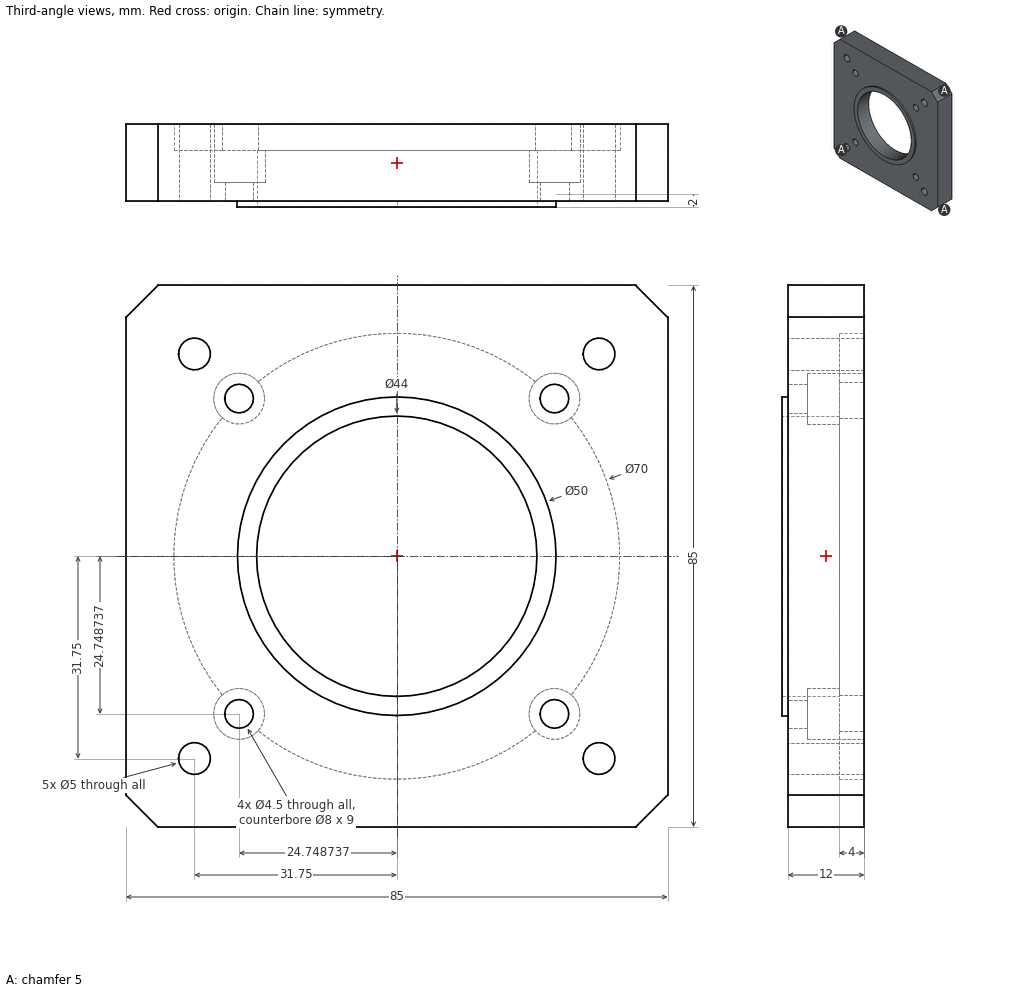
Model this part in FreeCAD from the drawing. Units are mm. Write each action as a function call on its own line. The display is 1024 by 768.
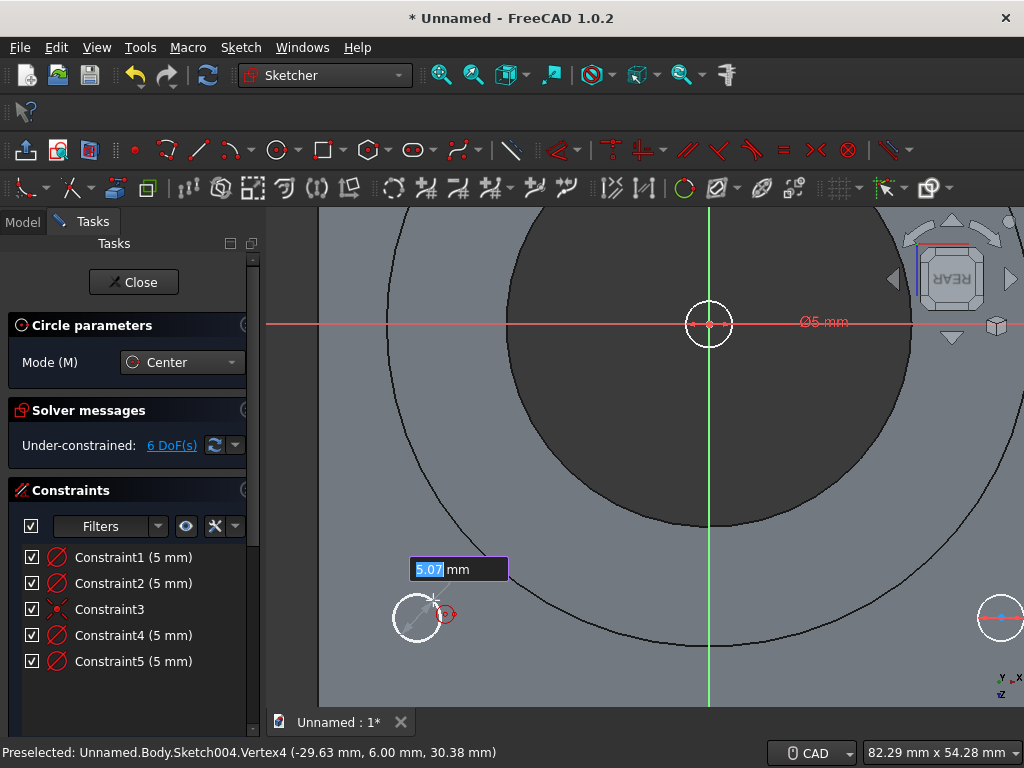
text(5)
key(Return)
key(Escape)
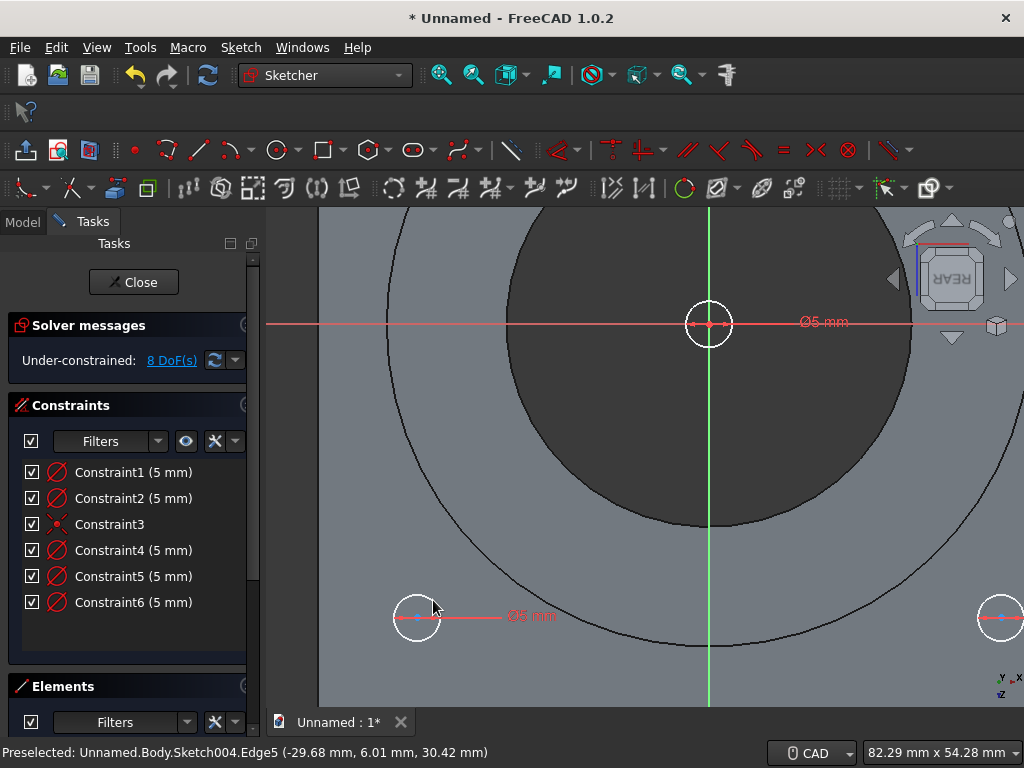
scroll(415, 618, down, 3)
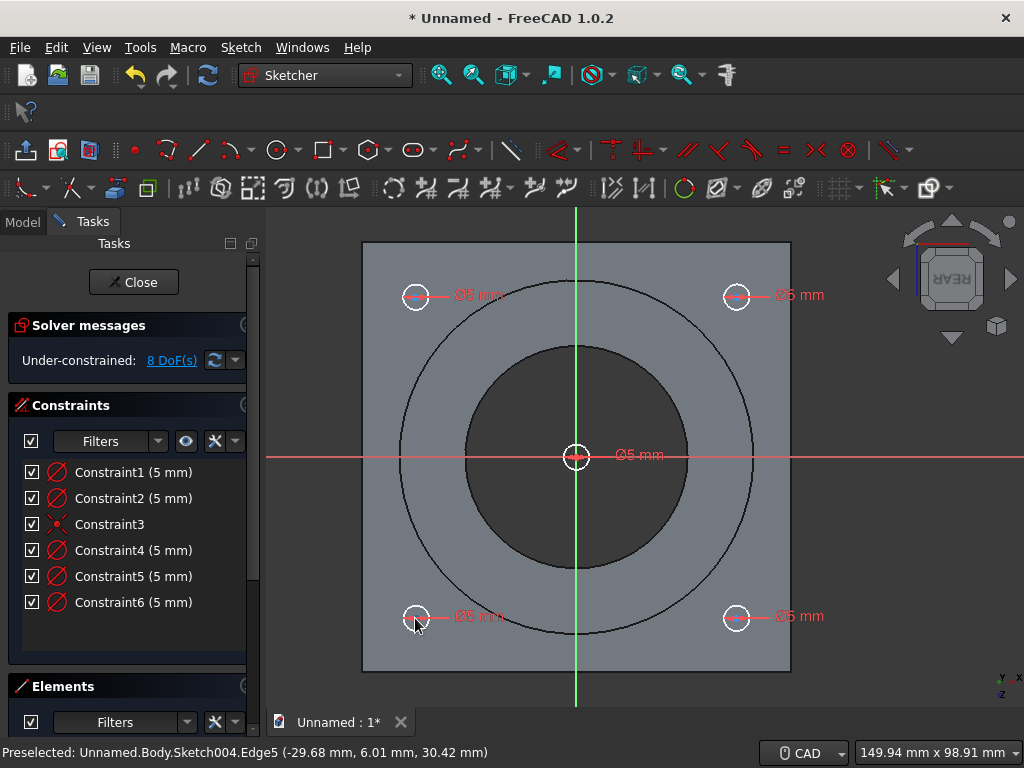
click(416, 297)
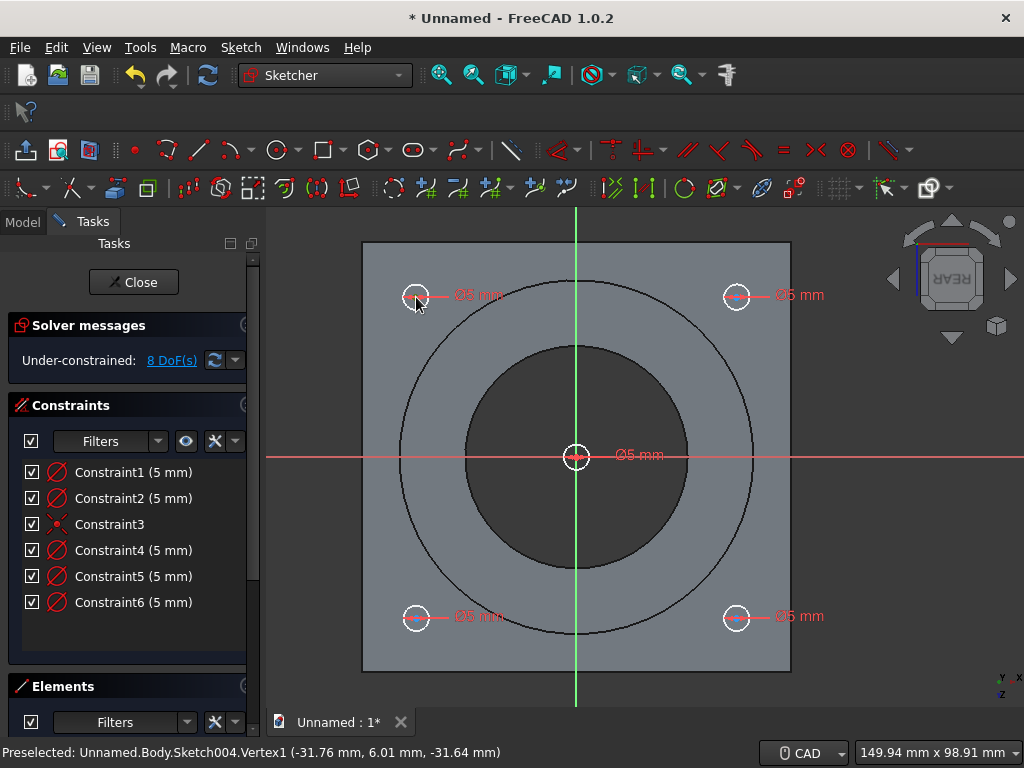
click(737, 297)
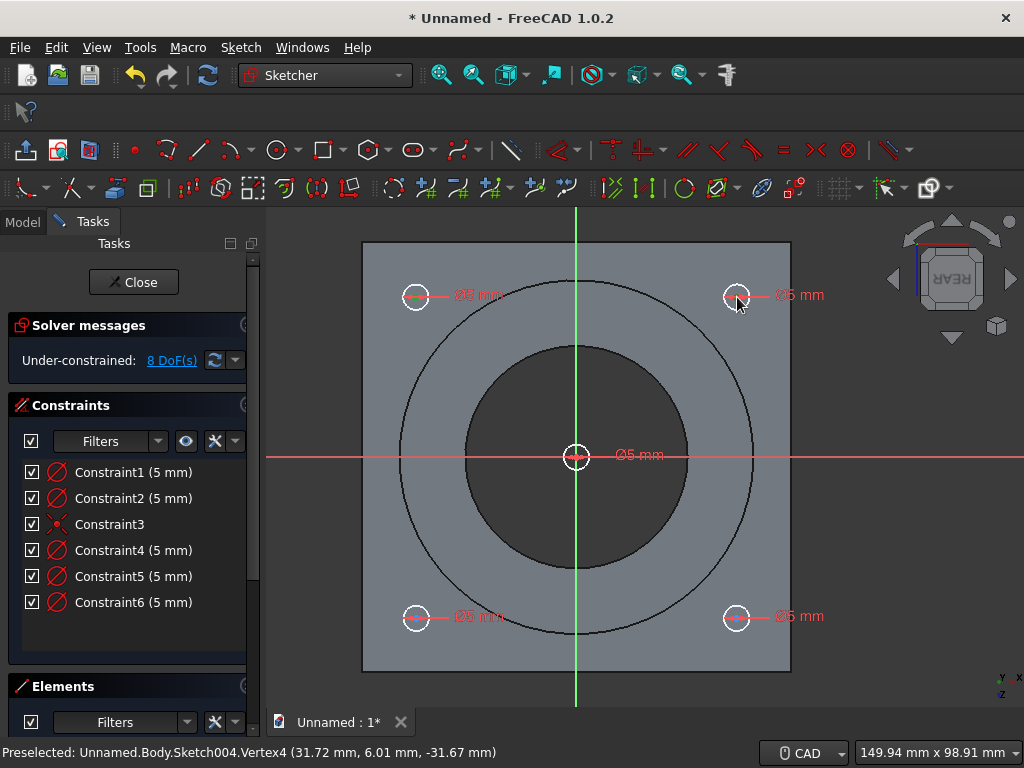
click(576, 647)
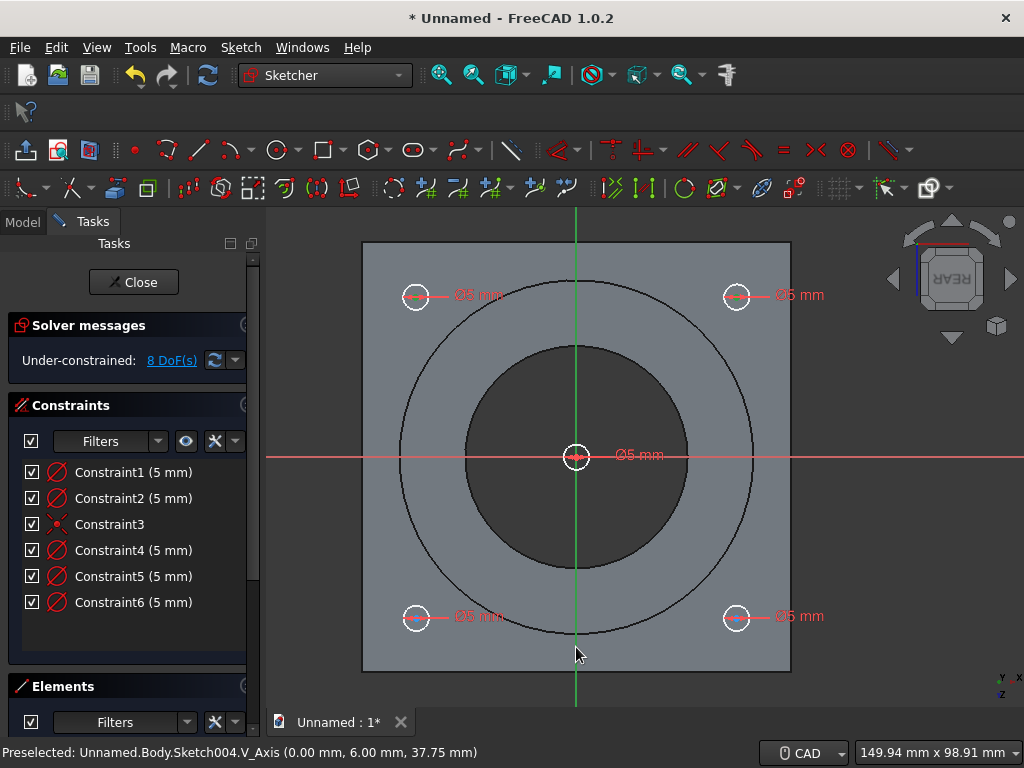
key(s)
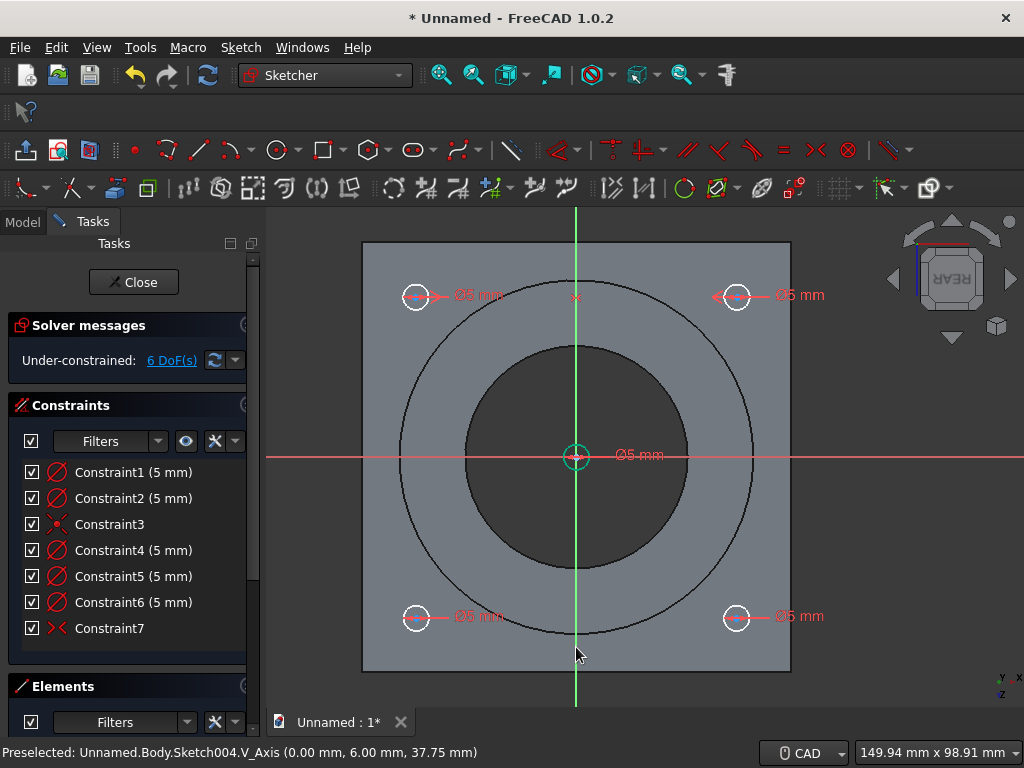
click(737, 618)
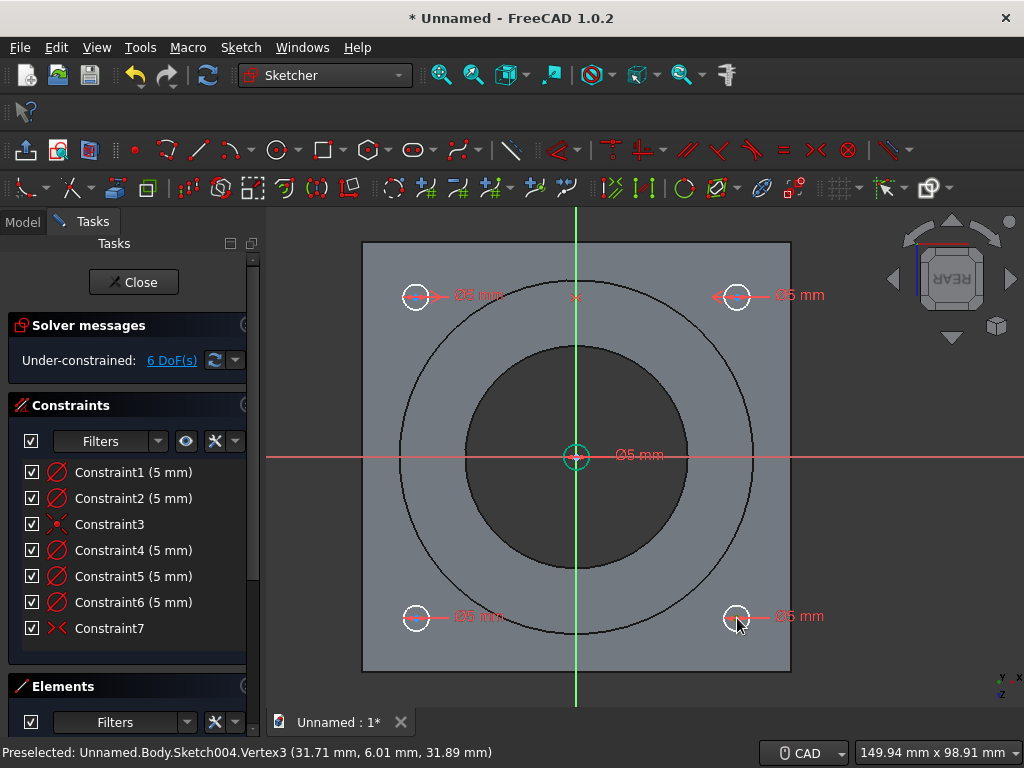
click(737, 297)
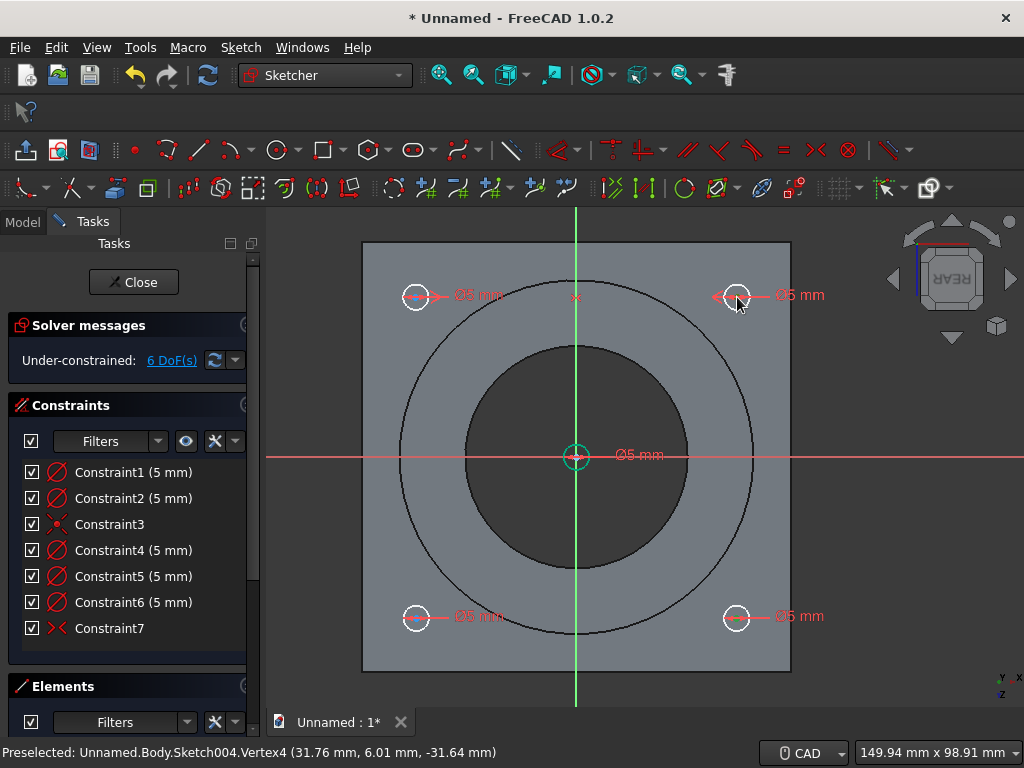
click(334, 457)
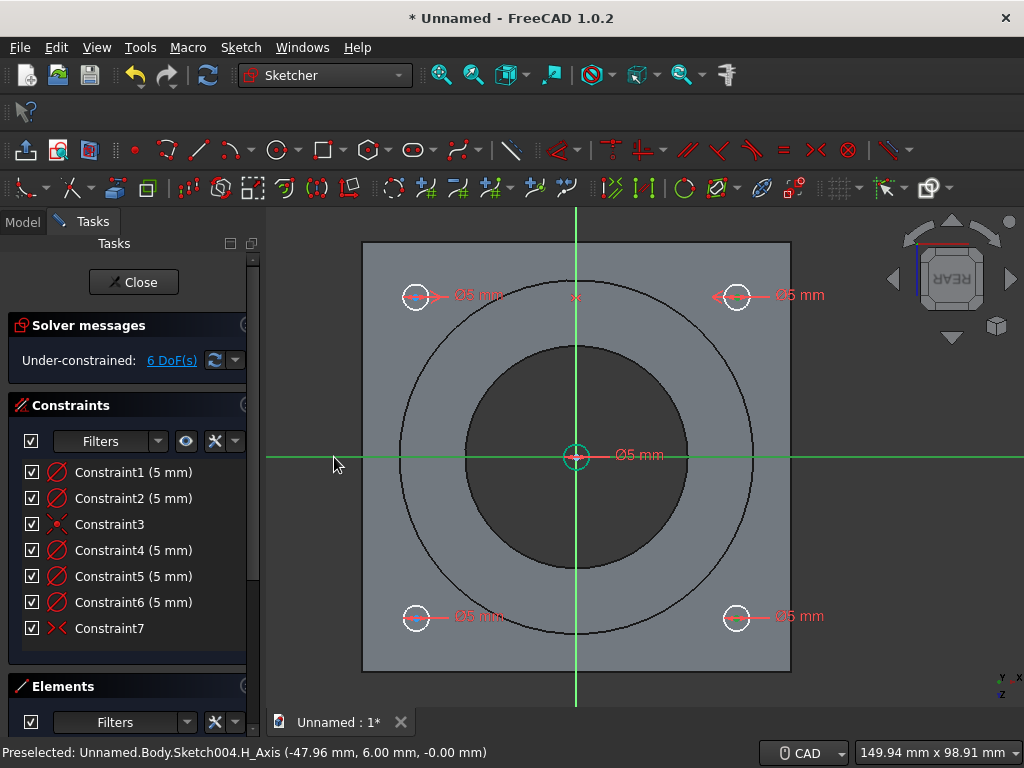
key(s)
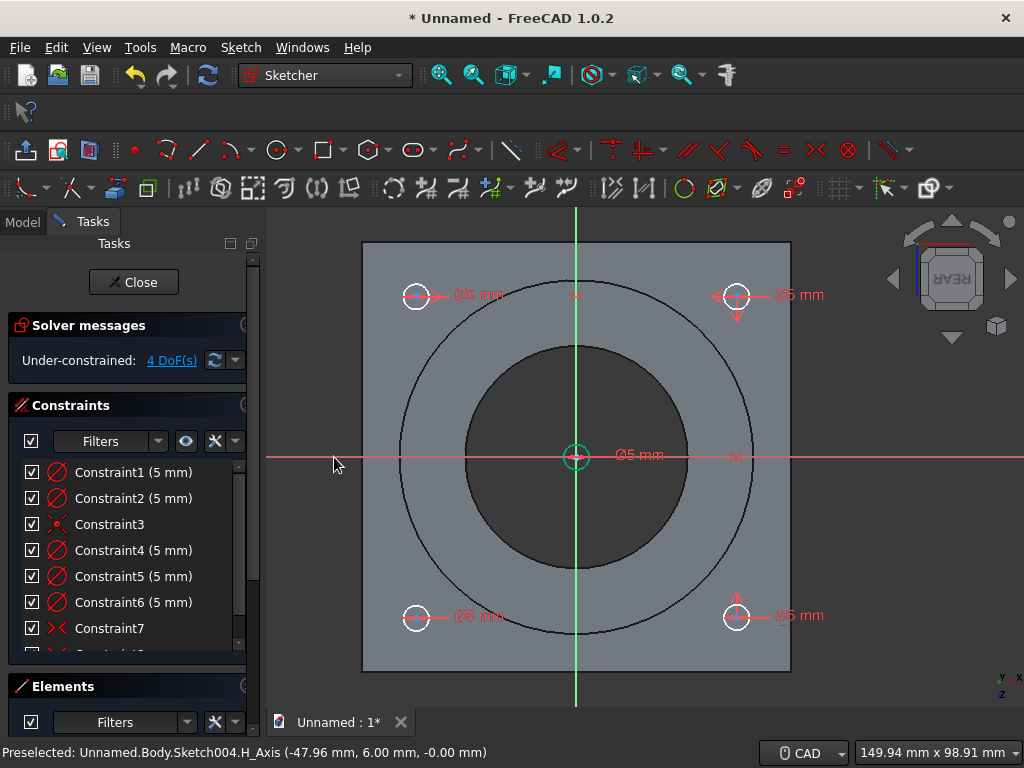
click(416, 297)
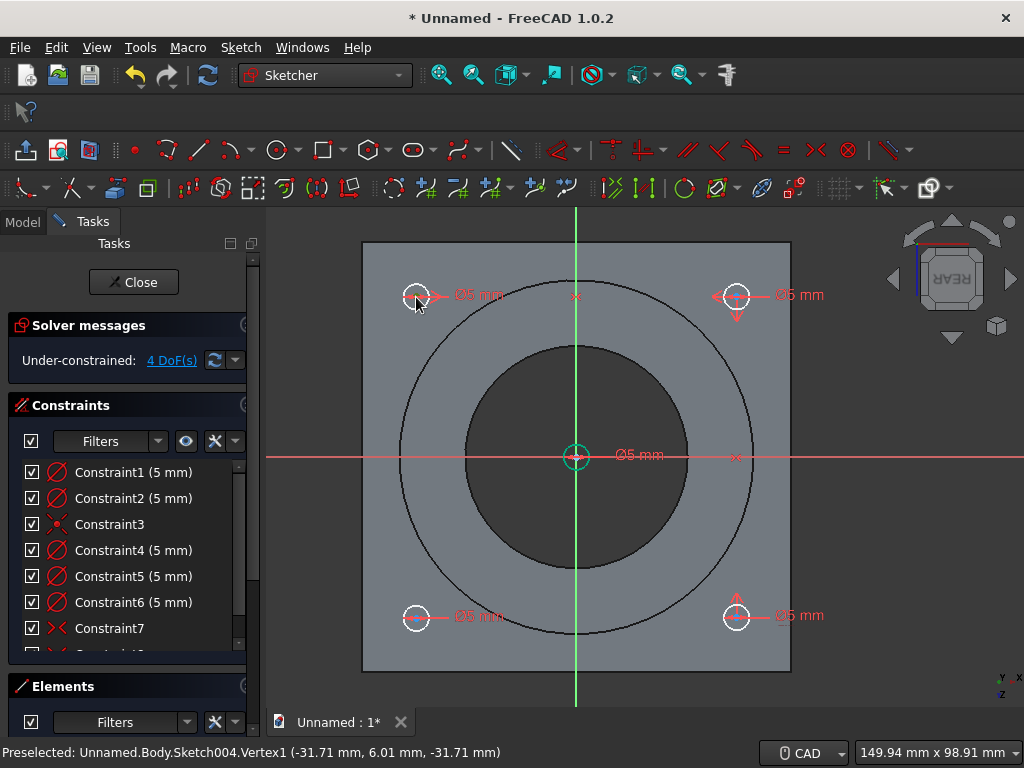
click(416, 618)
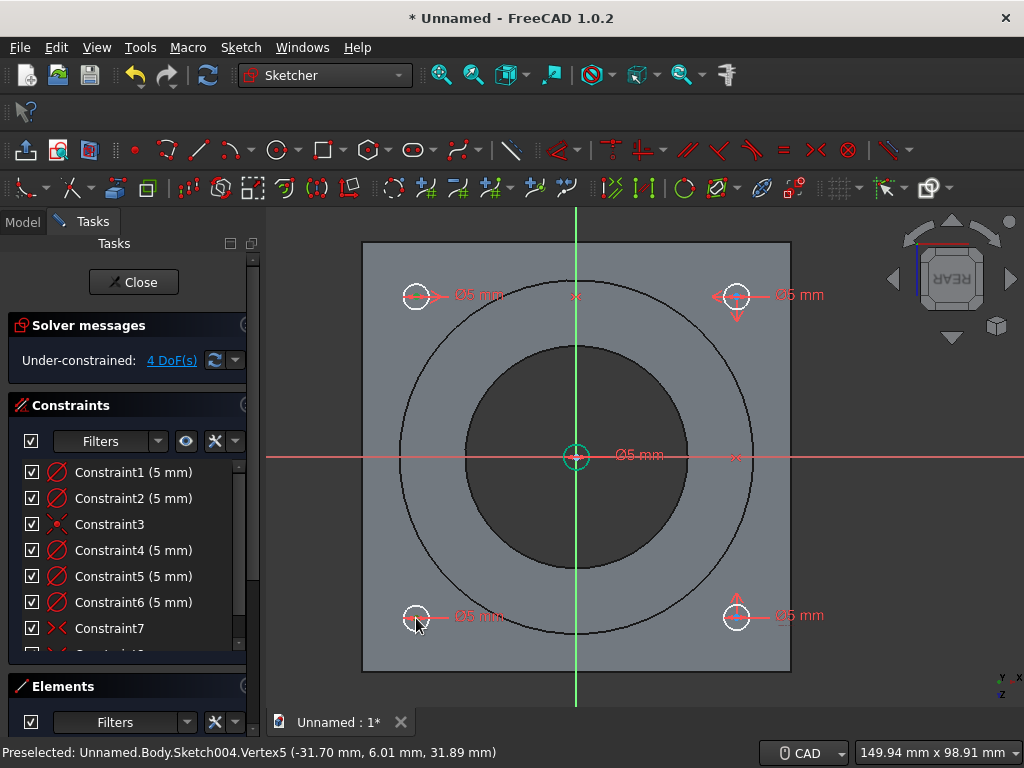
click(334, 457)